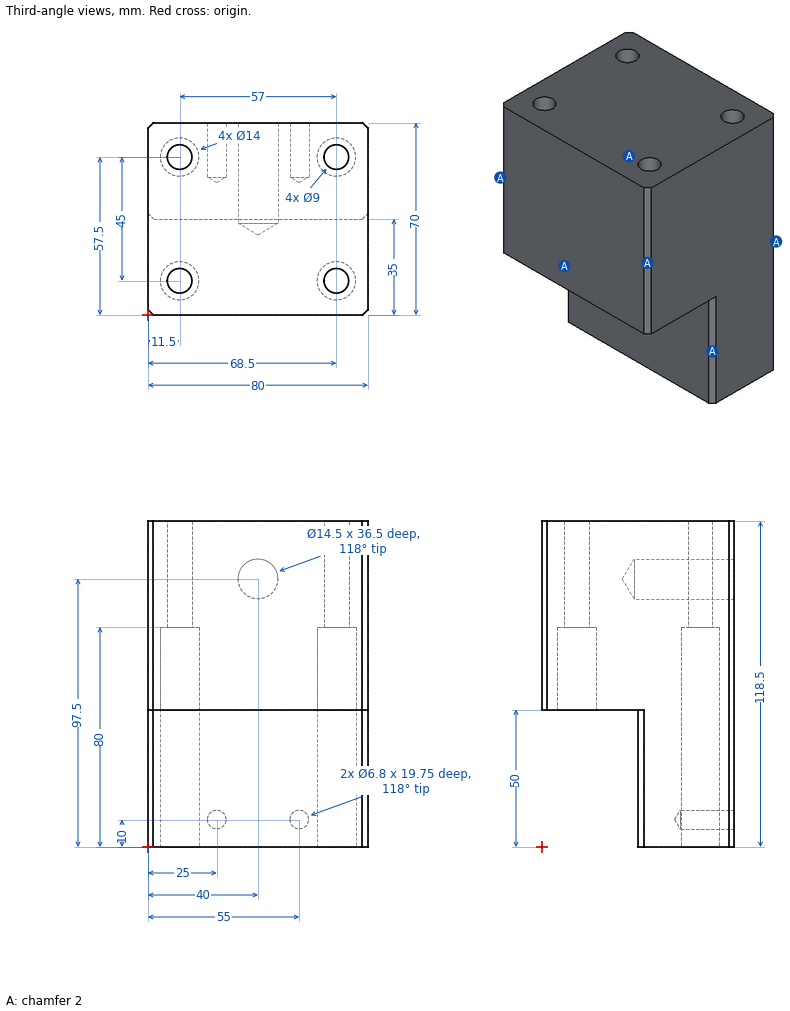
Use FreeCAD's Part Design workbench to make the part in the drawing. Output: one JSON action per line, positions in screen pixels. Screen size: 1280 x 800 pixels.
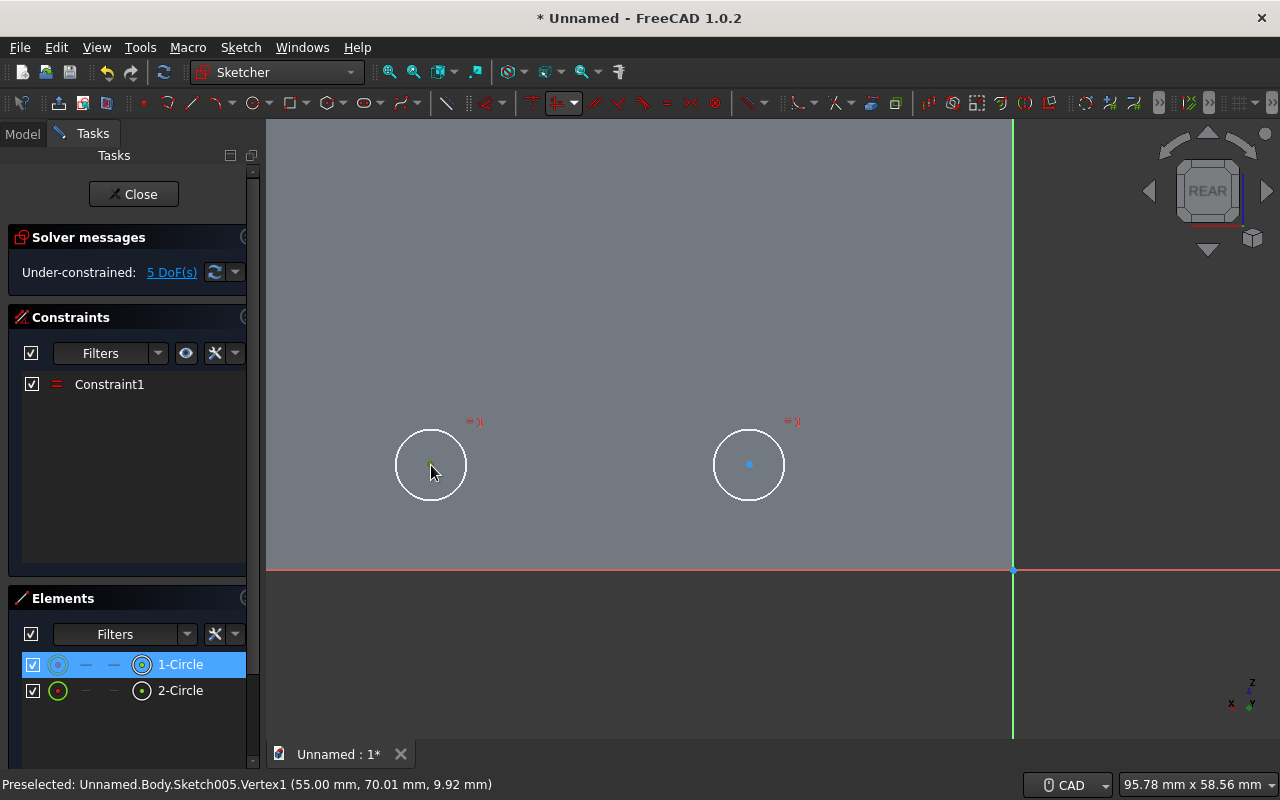
{"action": "left_click", "coordinate": [749, 465]}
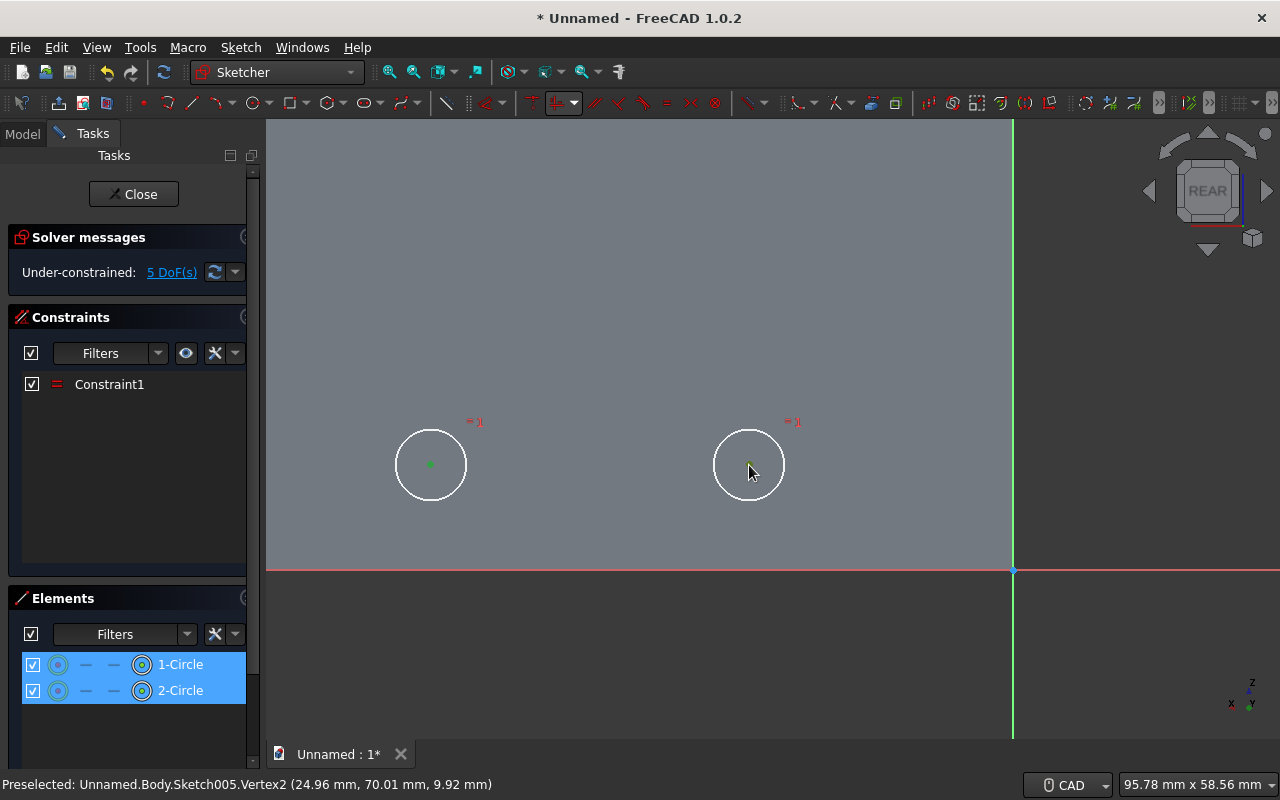
{"action": "key", "text": "h"}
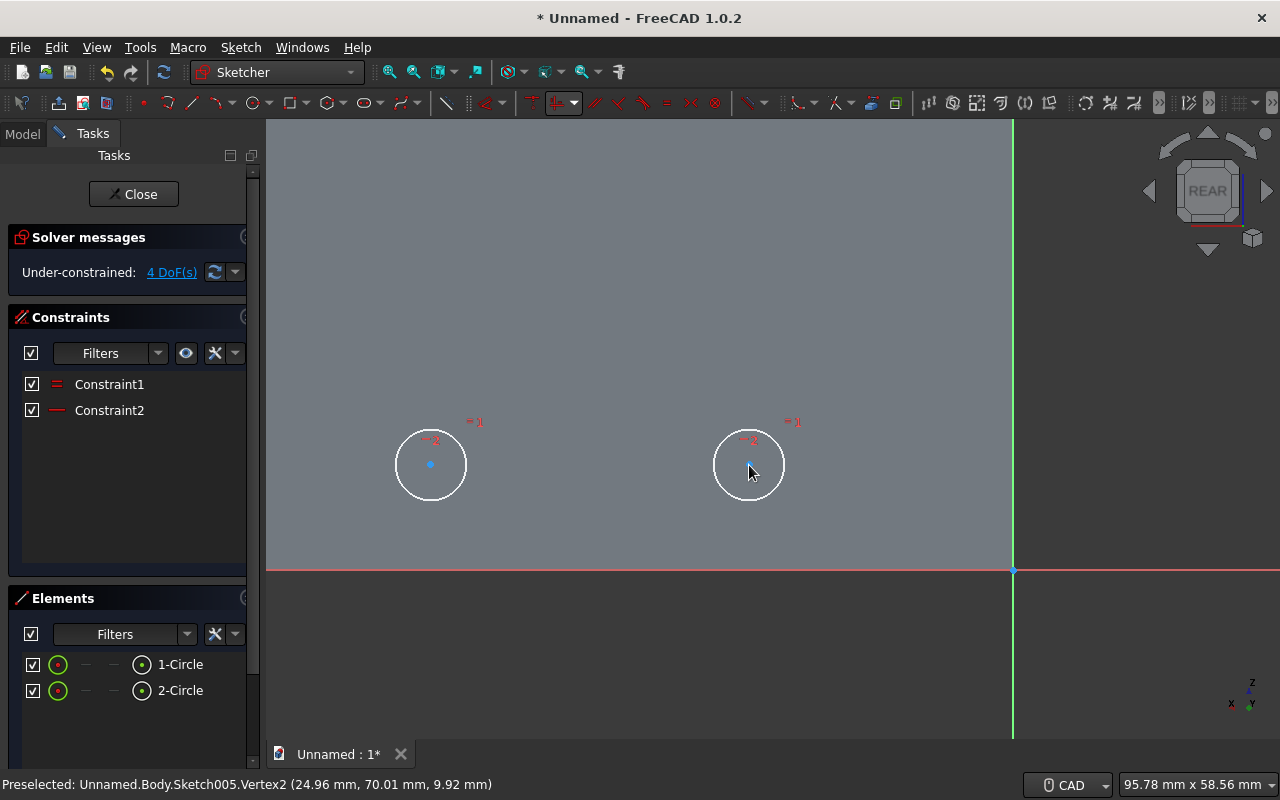
{"action": "left_click", "coordinate": [486, 104]}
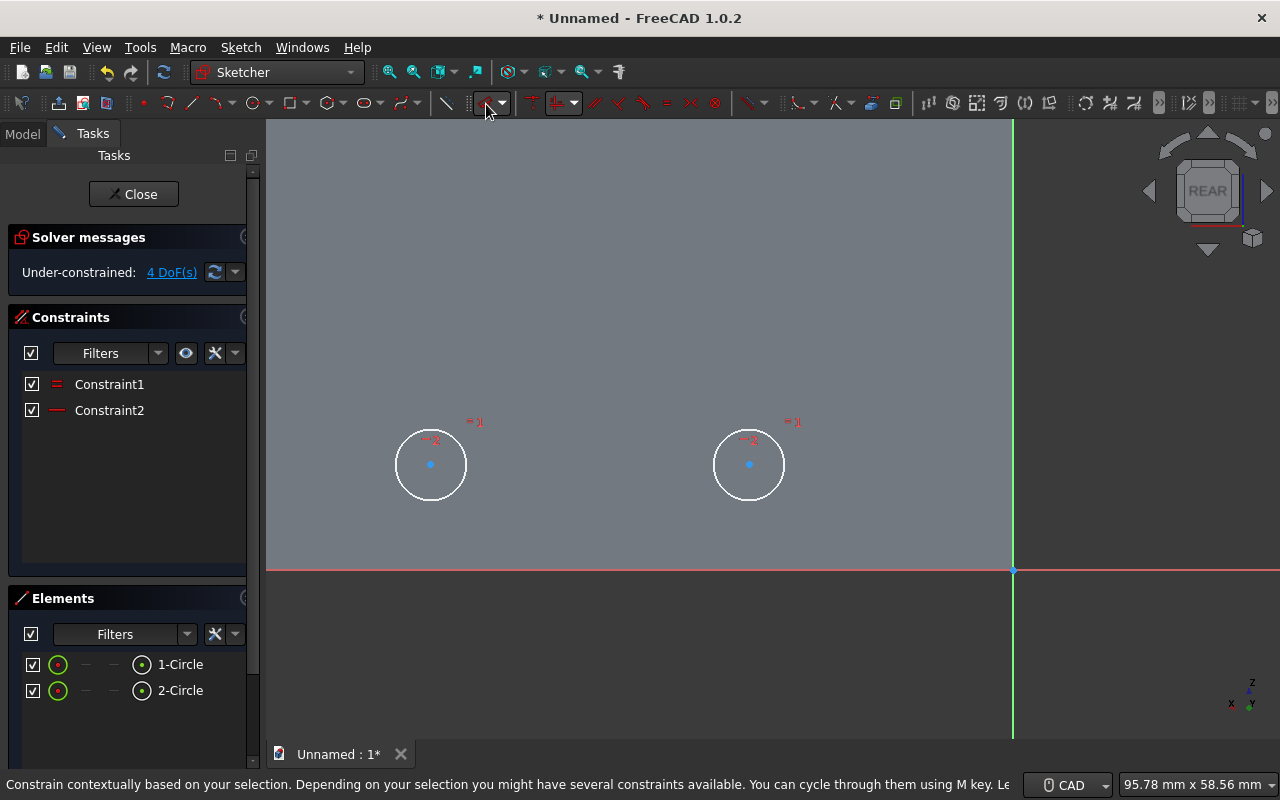
{"action": "left_click", "coordinate": [456, 440]}
{"action": "left_click", "coordinate": [479, 417]}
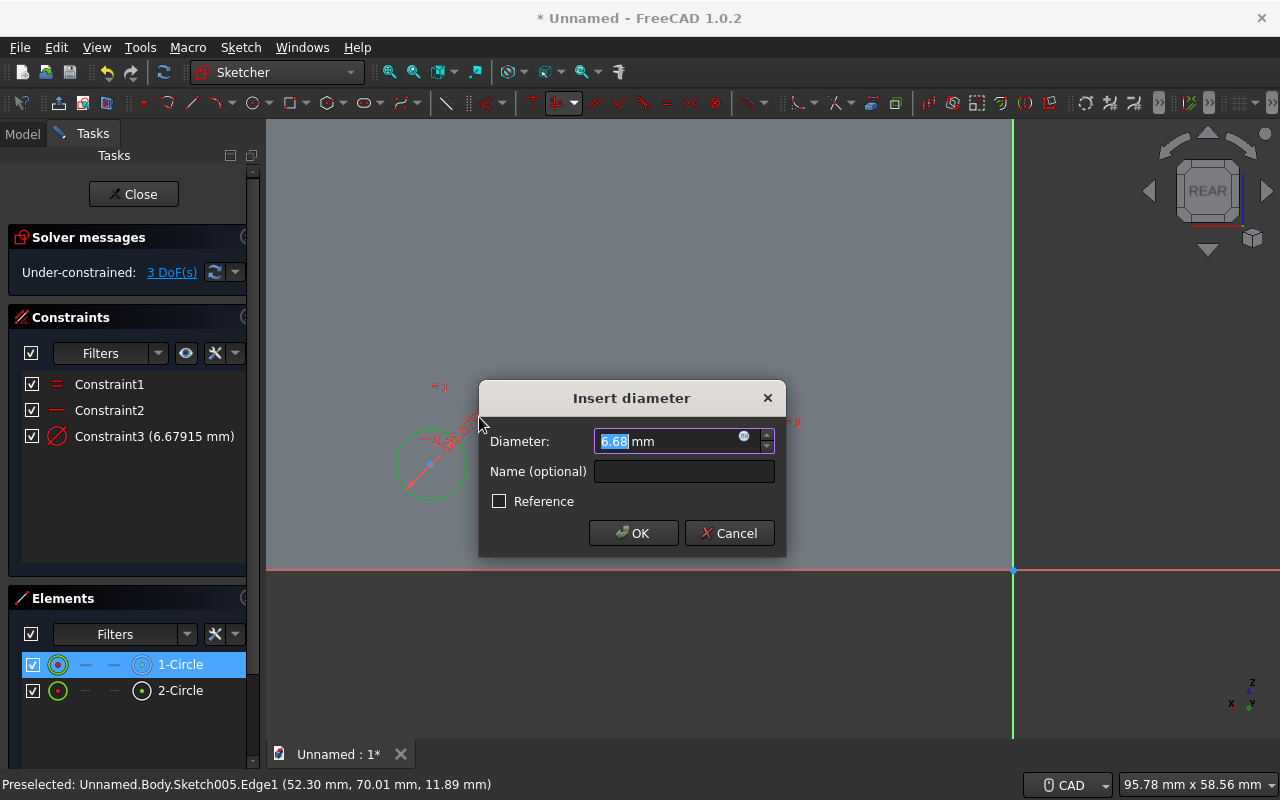
{"action": "type", "text": "6.8"}
{"action": "key", "text": "Return"}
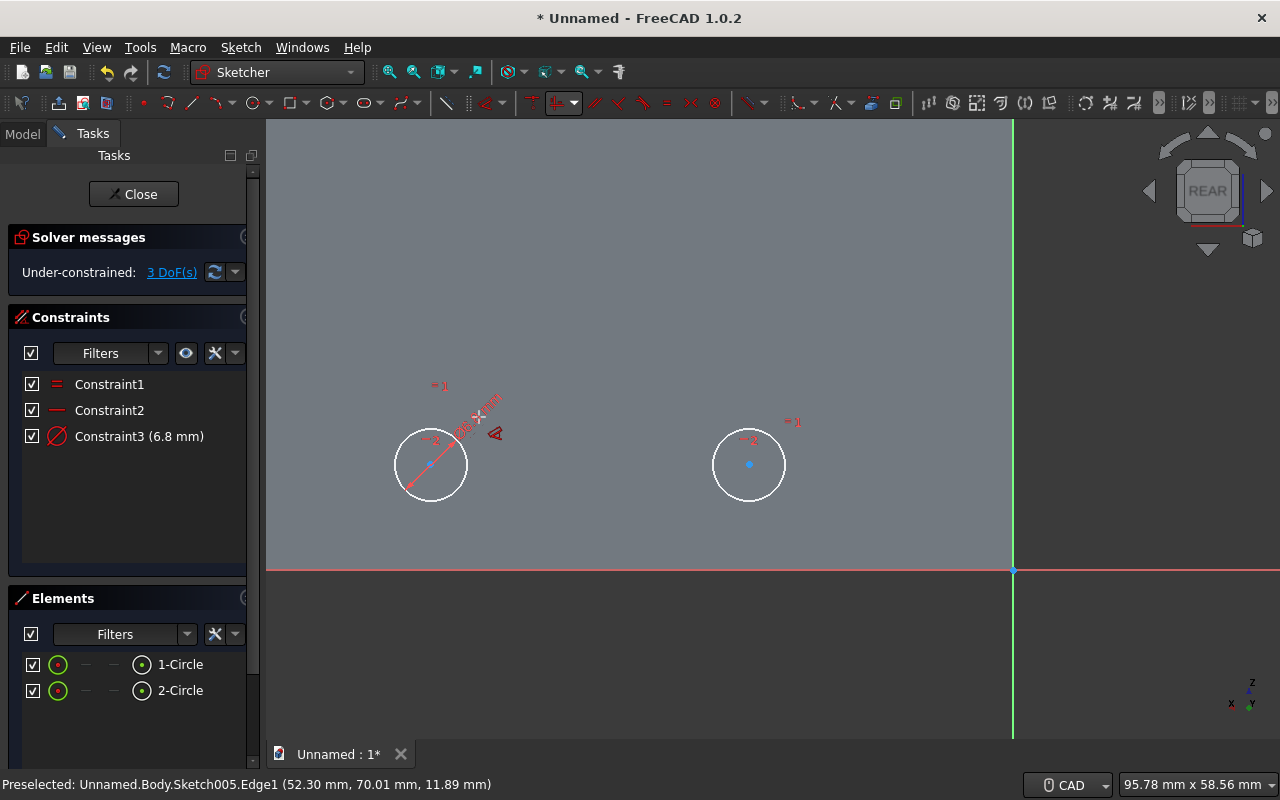
{"action": "left_click", "coordinate": [431, 465]}
{"action": "left_click", "coordinate": [722, 604]}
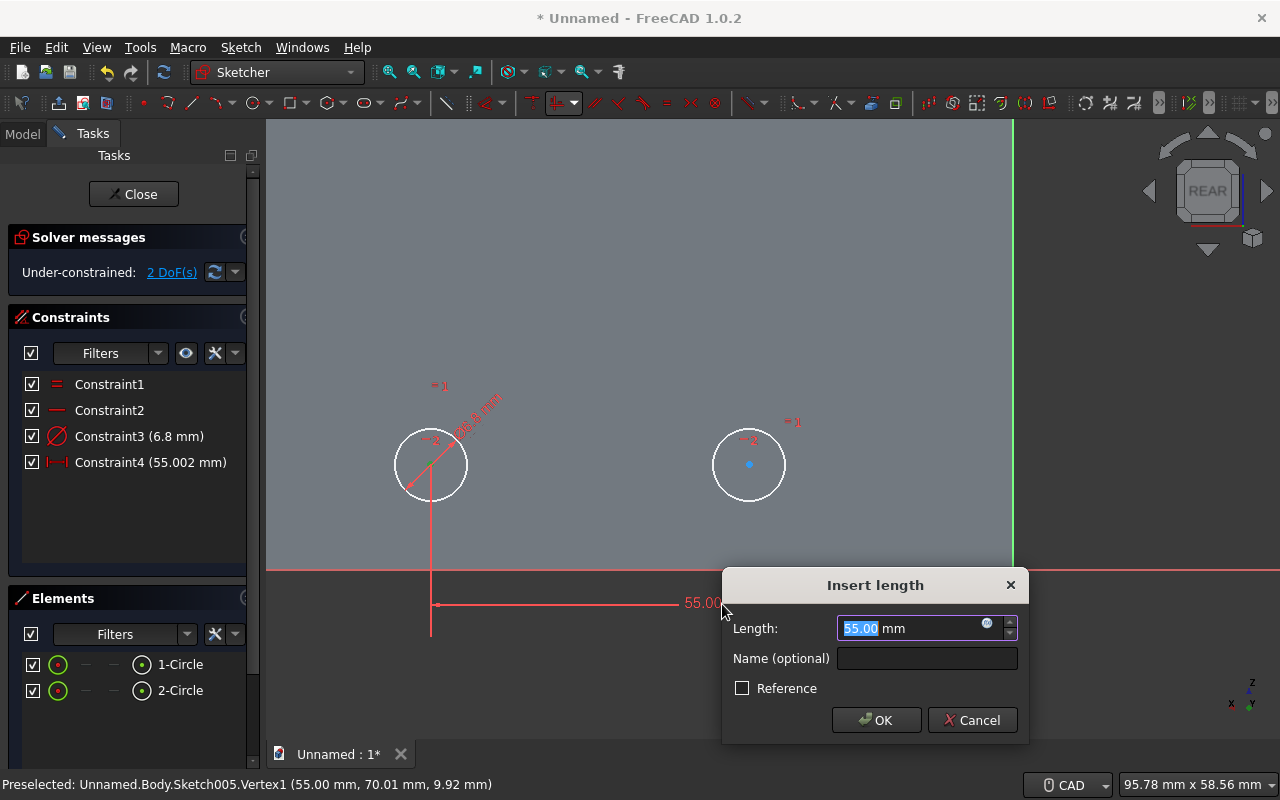
{"action": "type", "text": "55"}
{"action": "key", "text": "Return"}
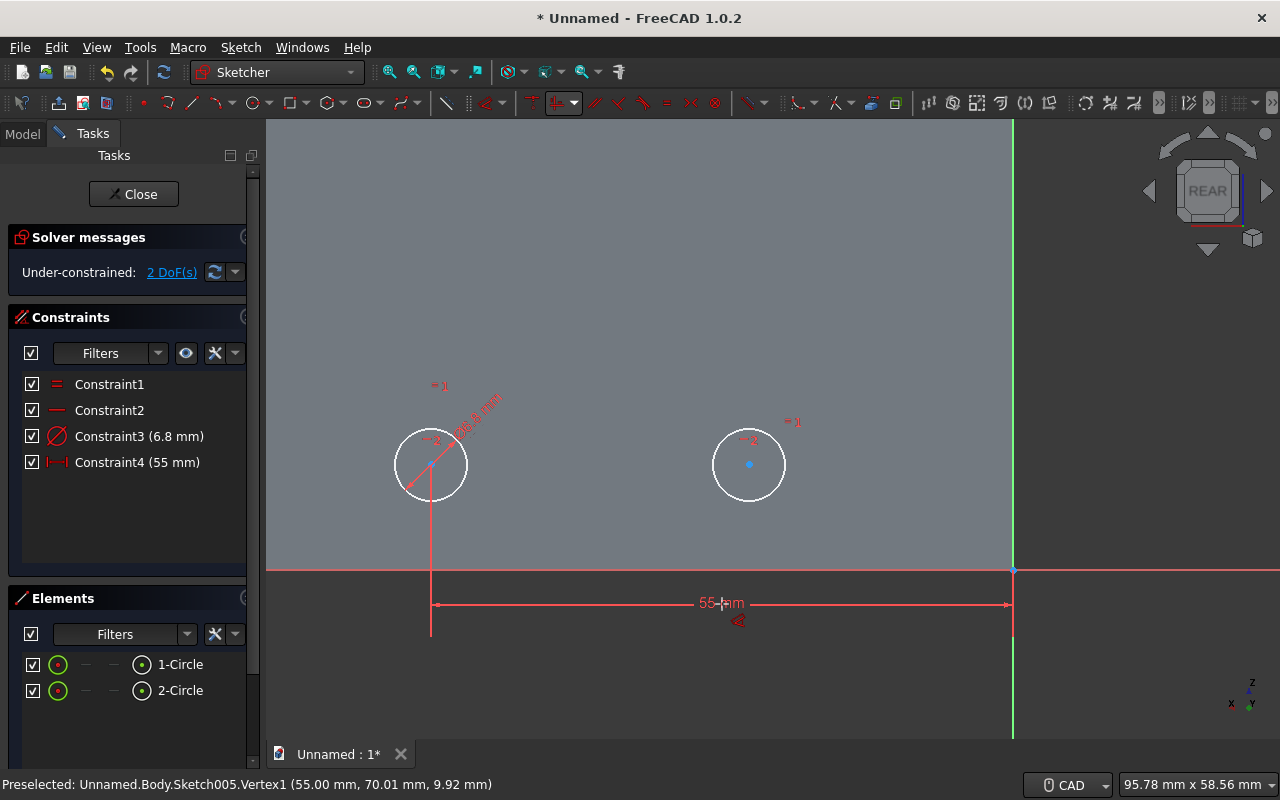
{"action": "left_click", "coordinate": [431, 465]}
{"action": "left_click", "coordinate": [1047, 518]}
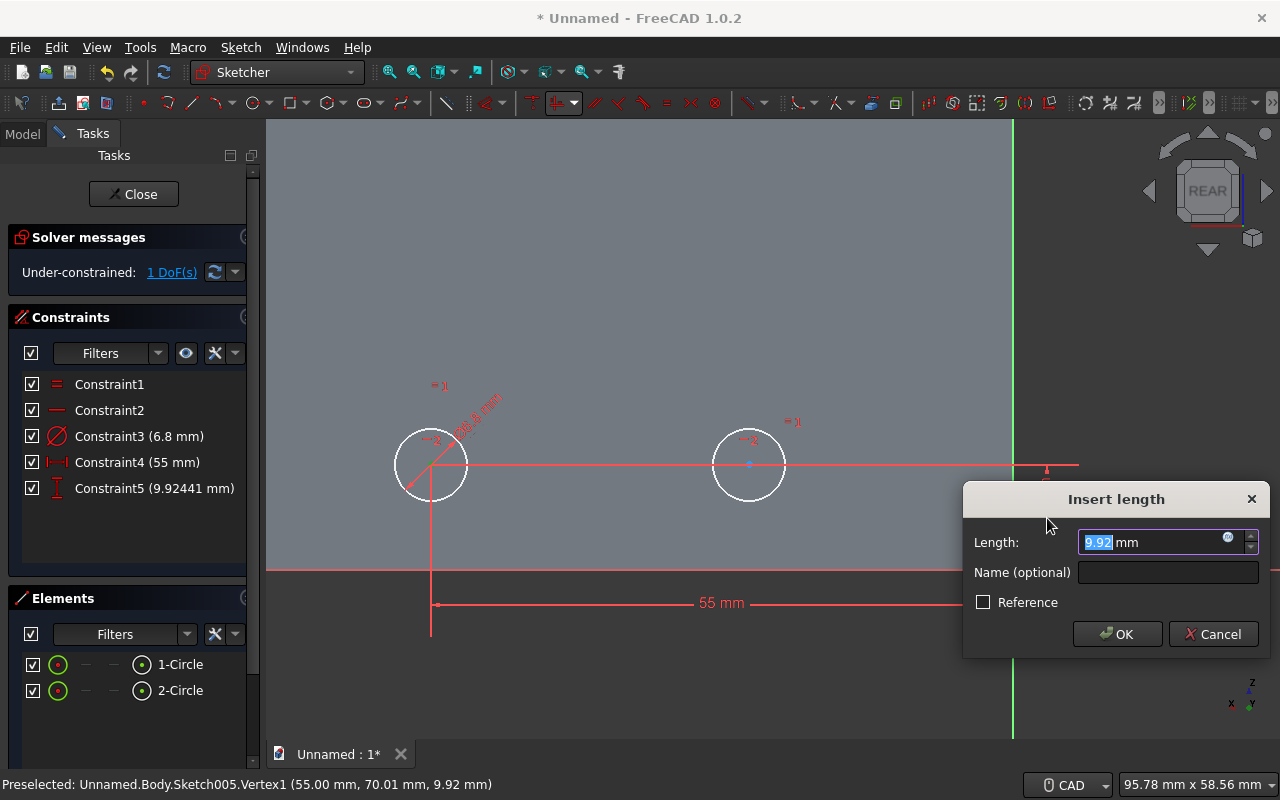
{"action": "type", "text": "10"}
{"action": "key", "text": "Return"}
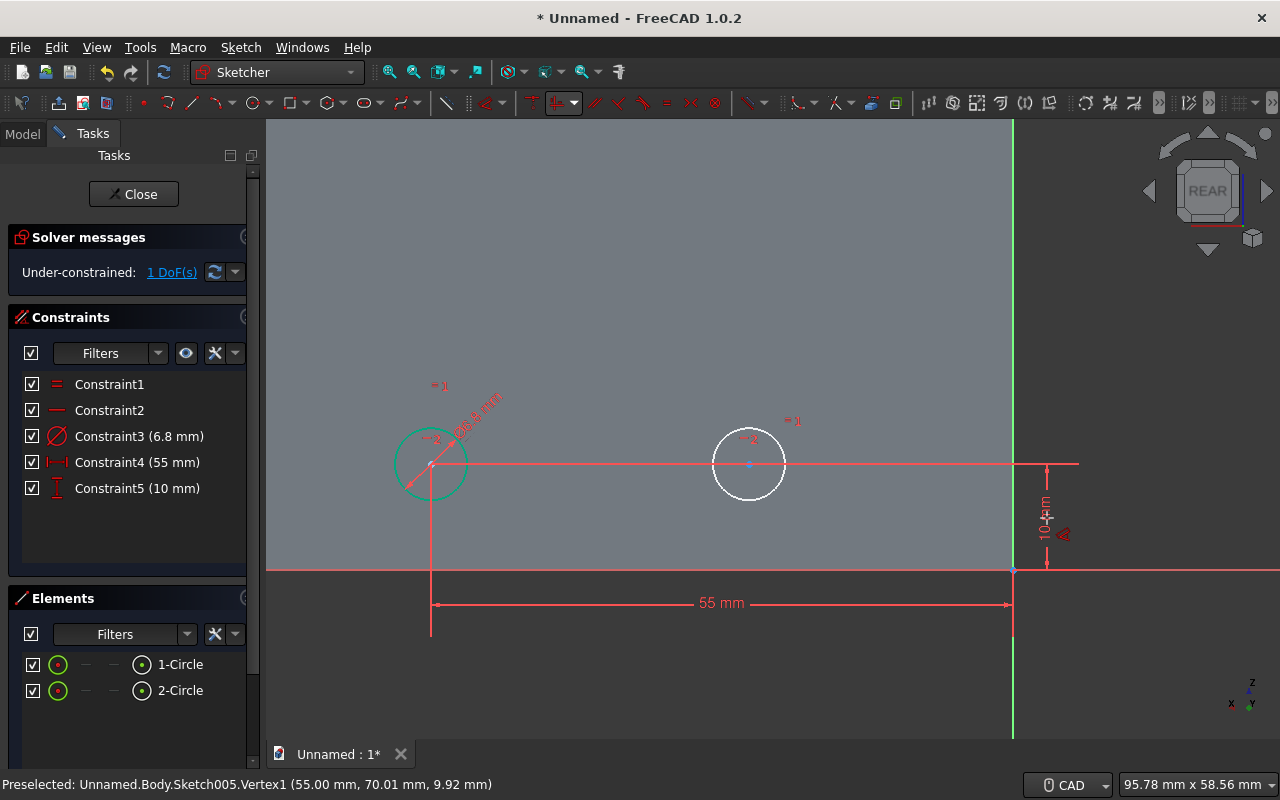
{"action": "left_click", "coordinate": [749, 464]}
{"action": "left_click", "coordinate": [881, 604]}